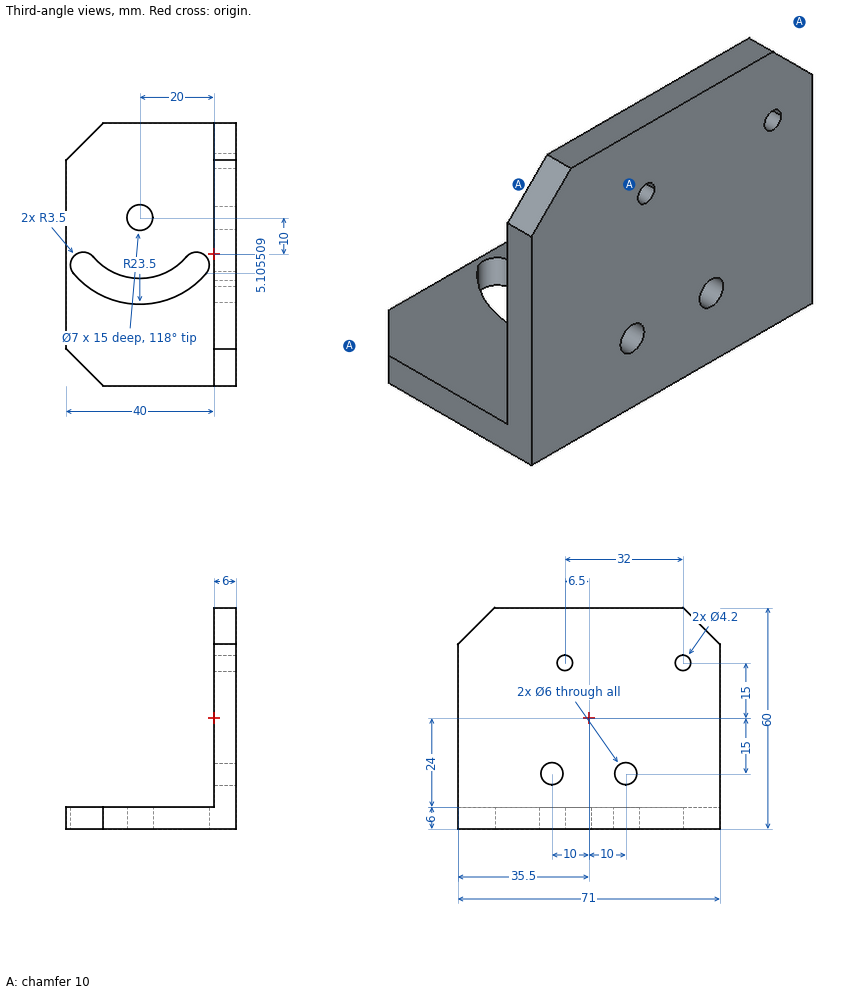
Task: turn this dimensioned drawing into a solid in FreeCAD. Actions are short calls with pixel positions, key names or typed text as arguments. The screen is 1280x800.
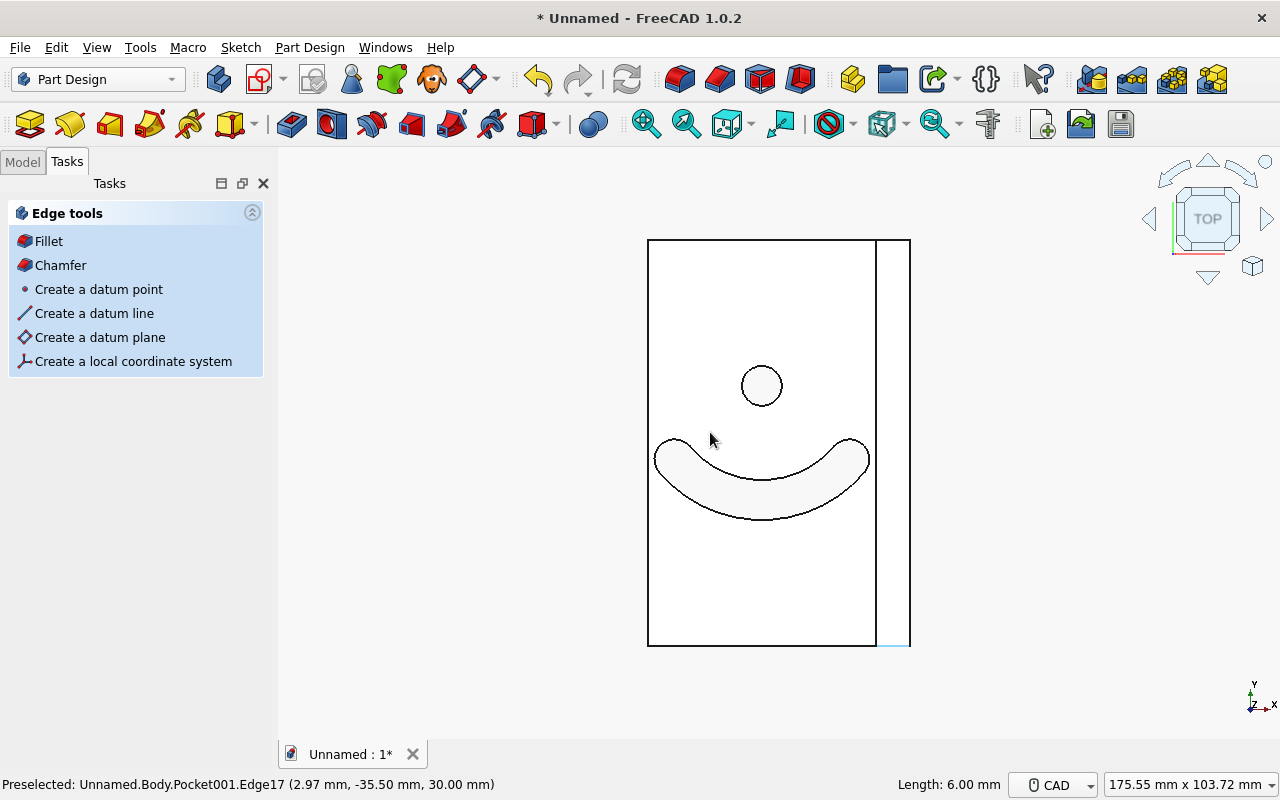
click(893, 239, ctrl)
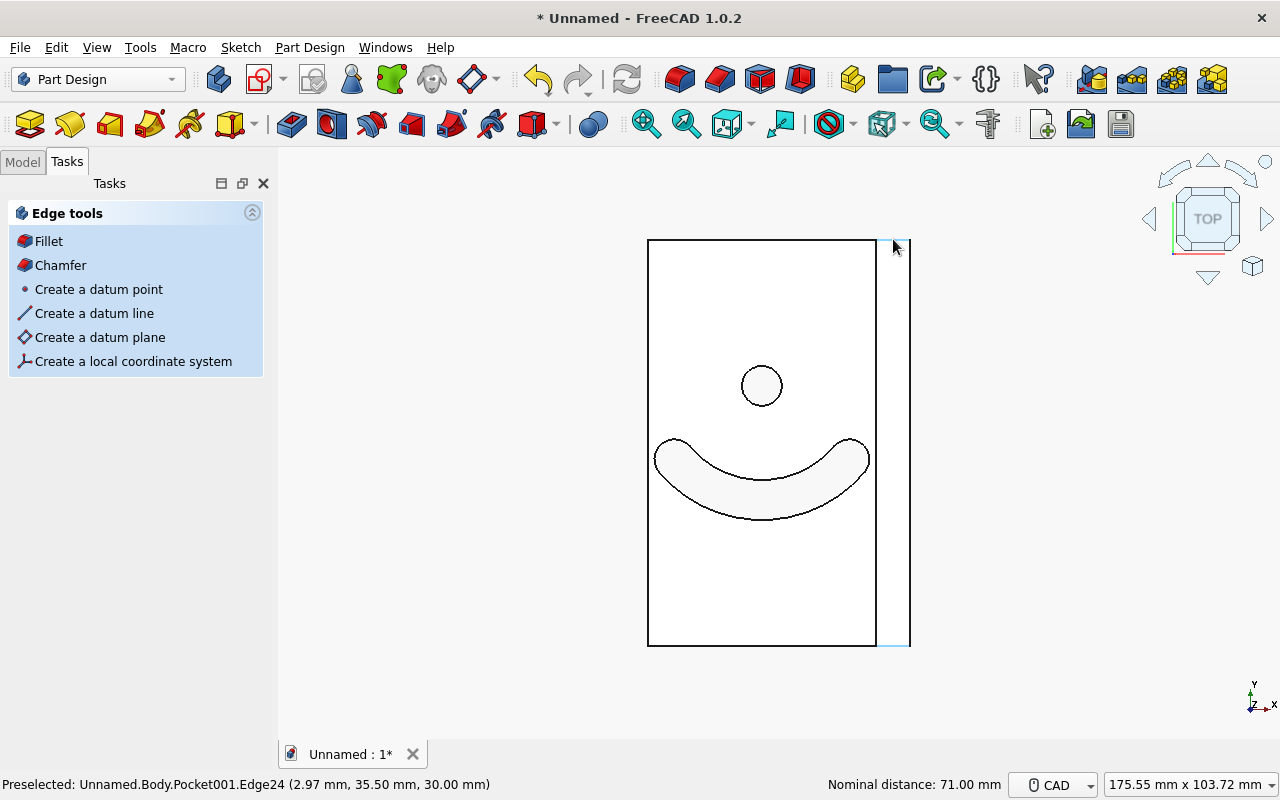
key(1)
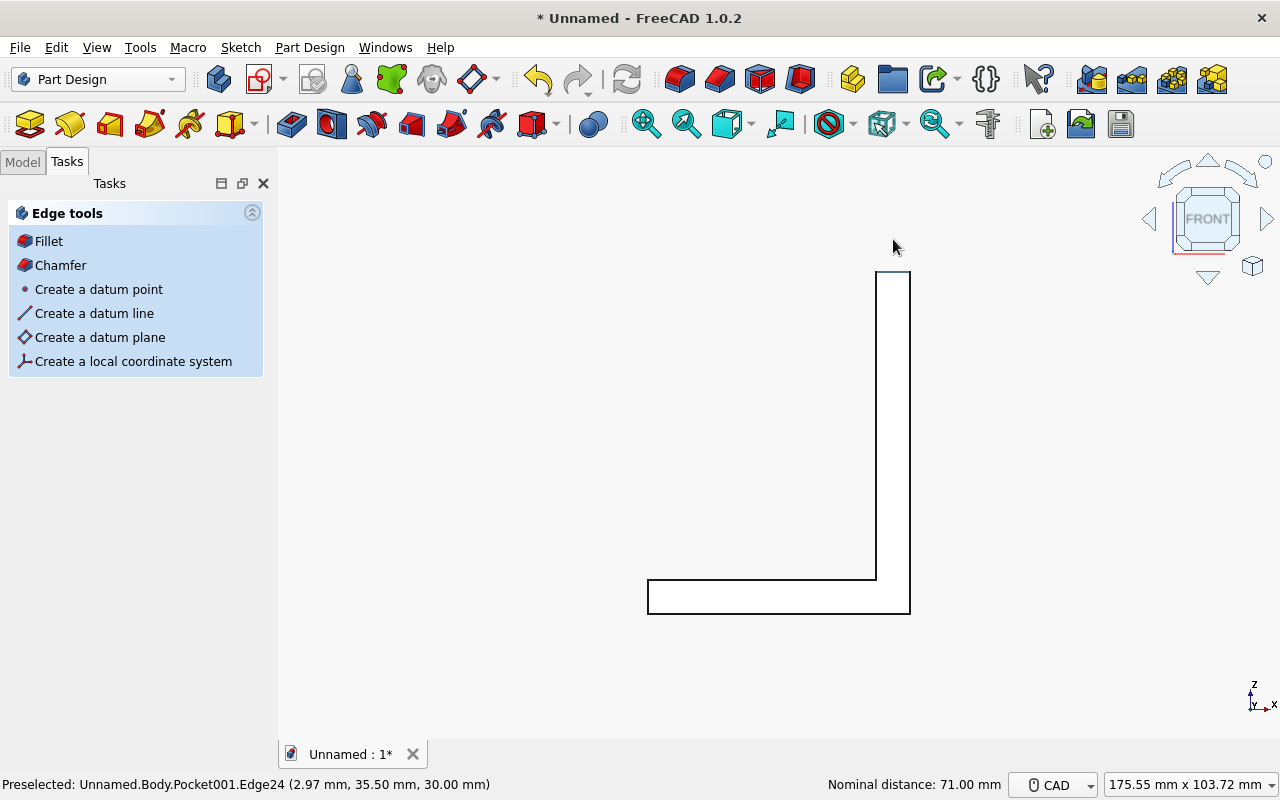
click(648, 596, ctrl)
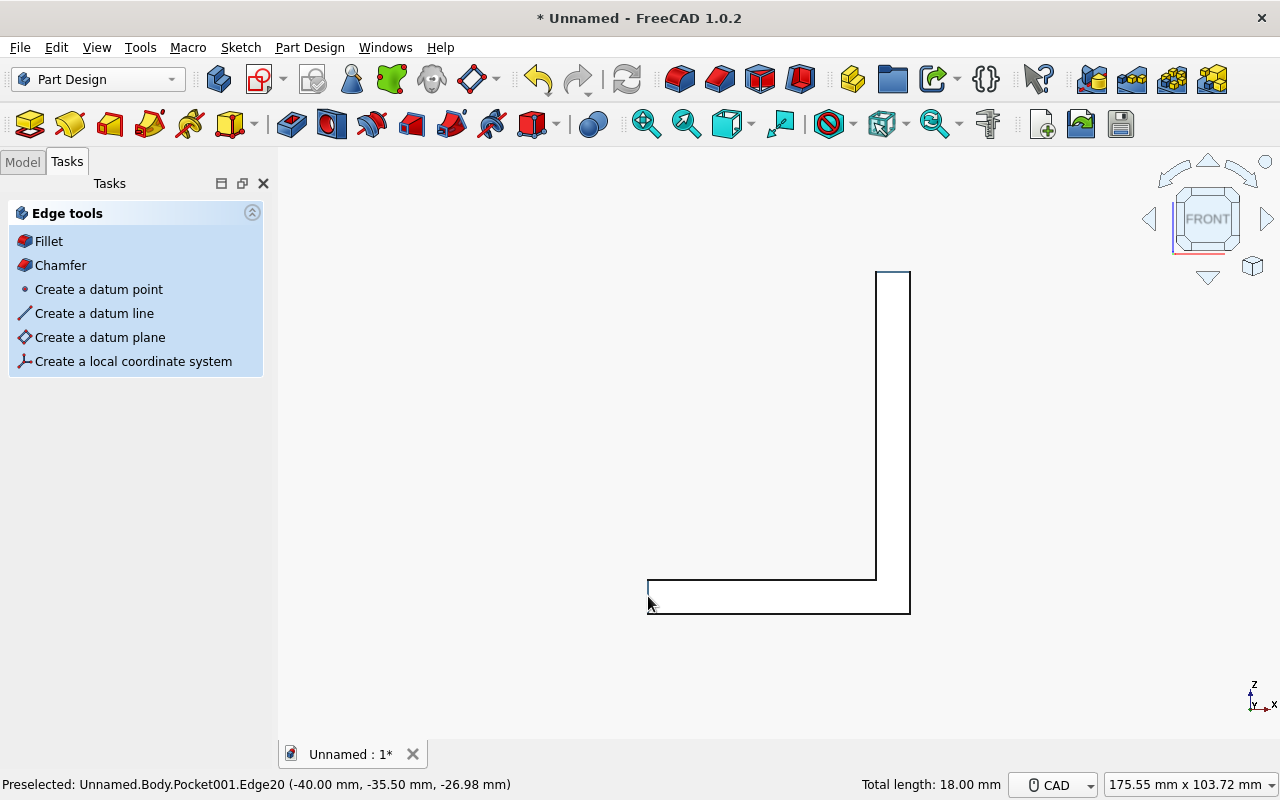
key(3)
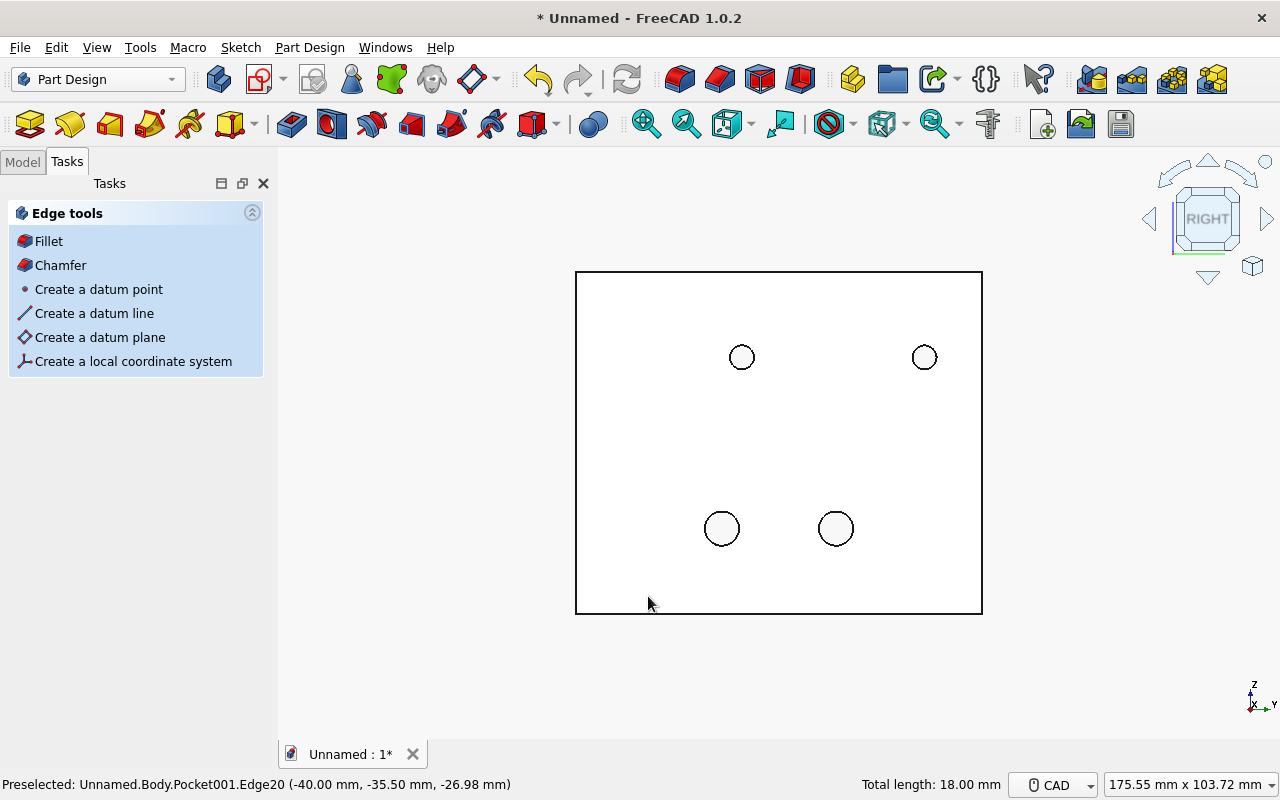
key(5)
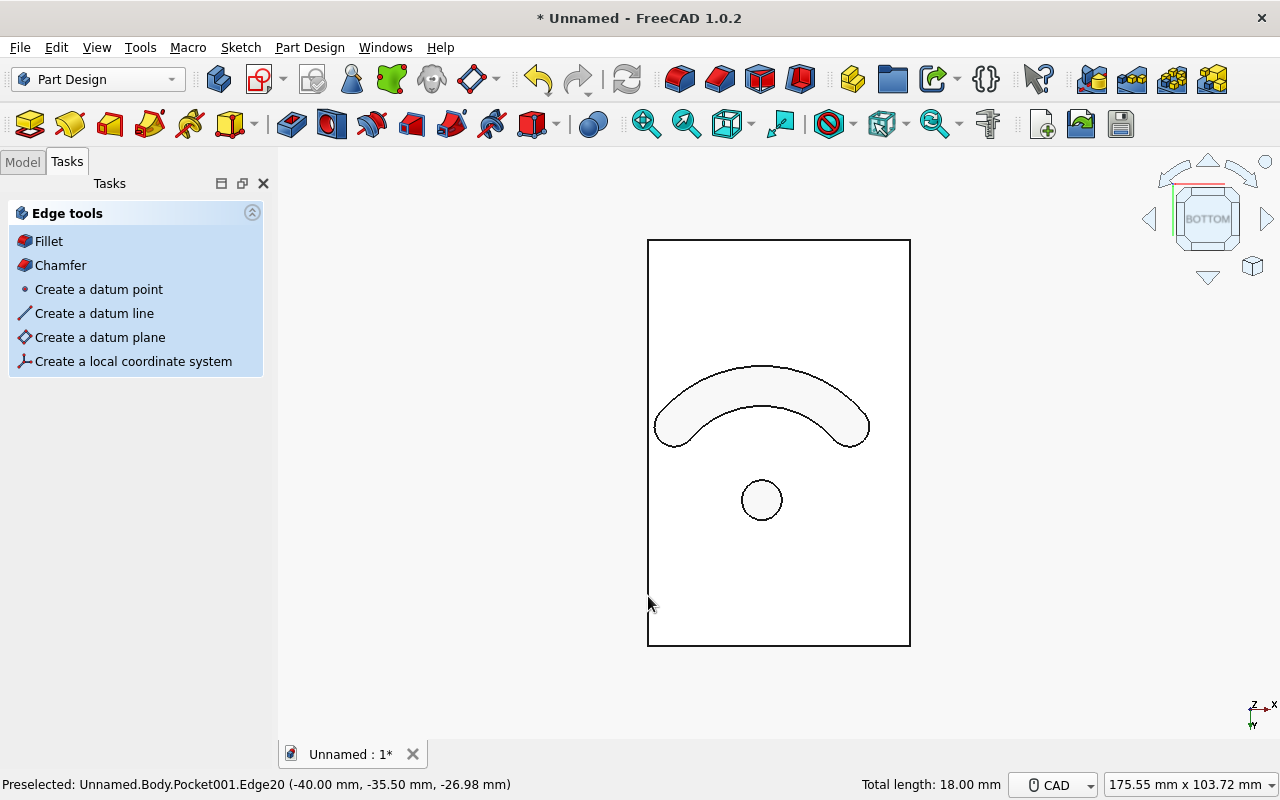
key(4)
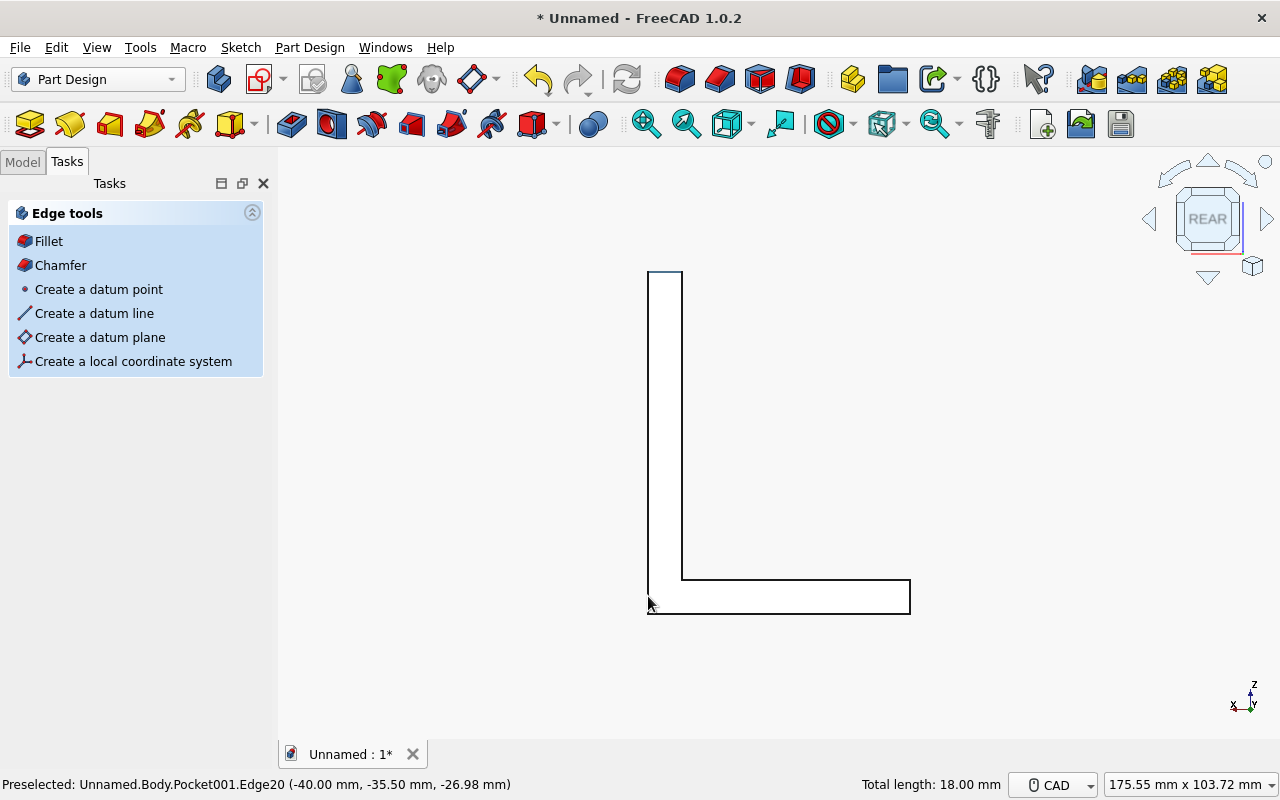
click(910, 596, ctrl)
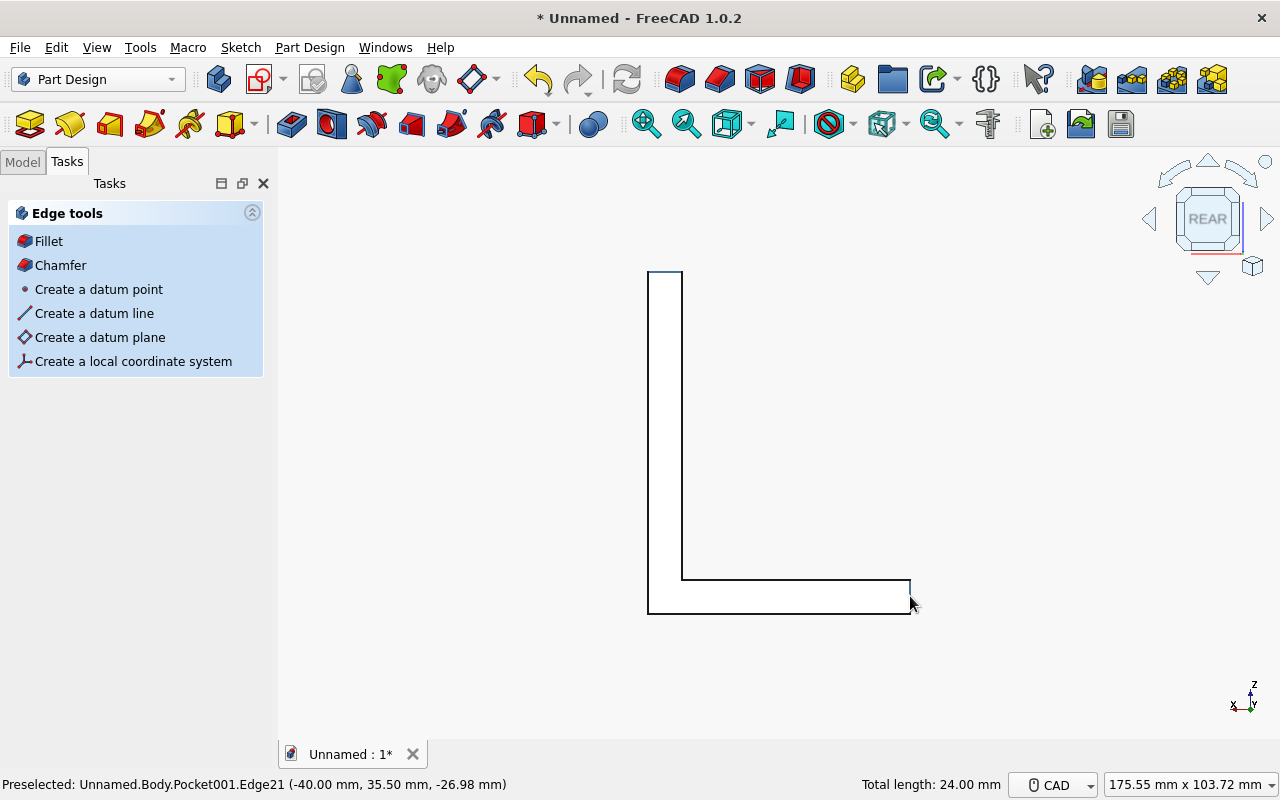
click(720, 80)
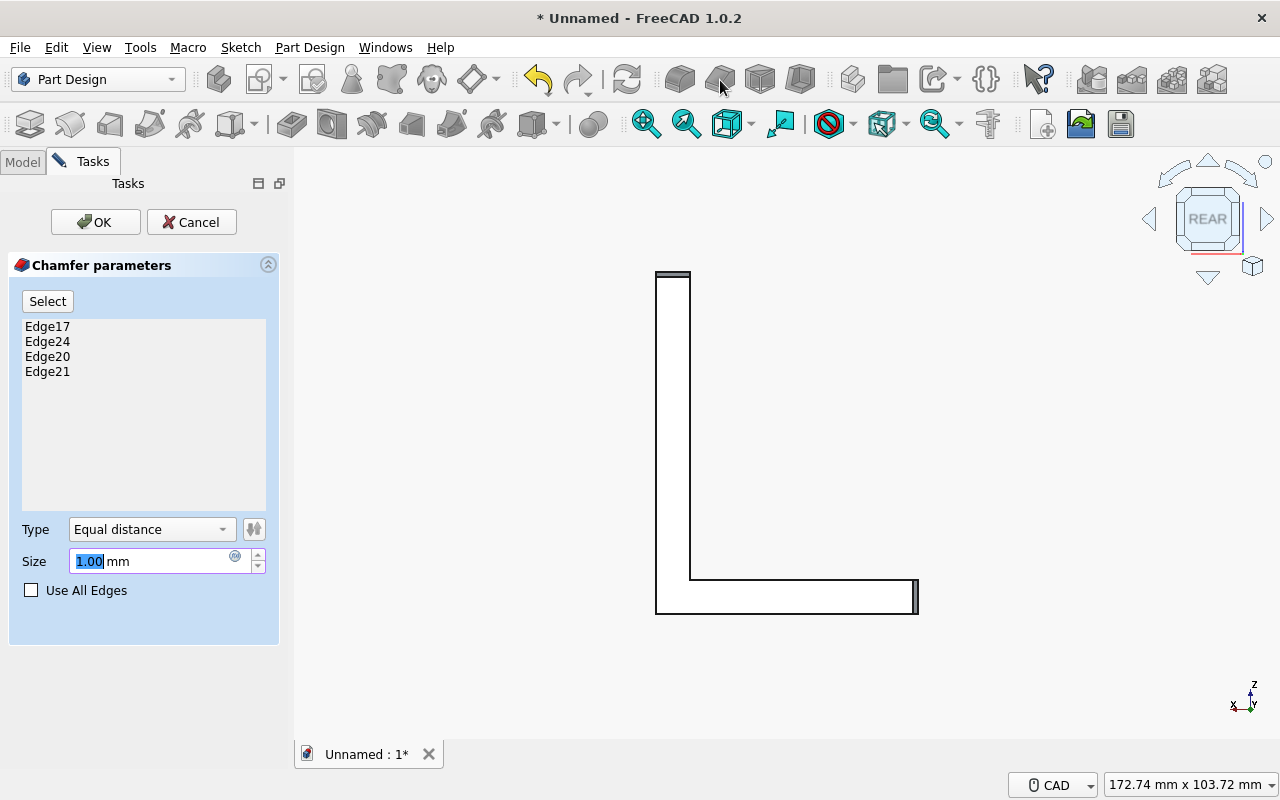
text(10)
key(Tab)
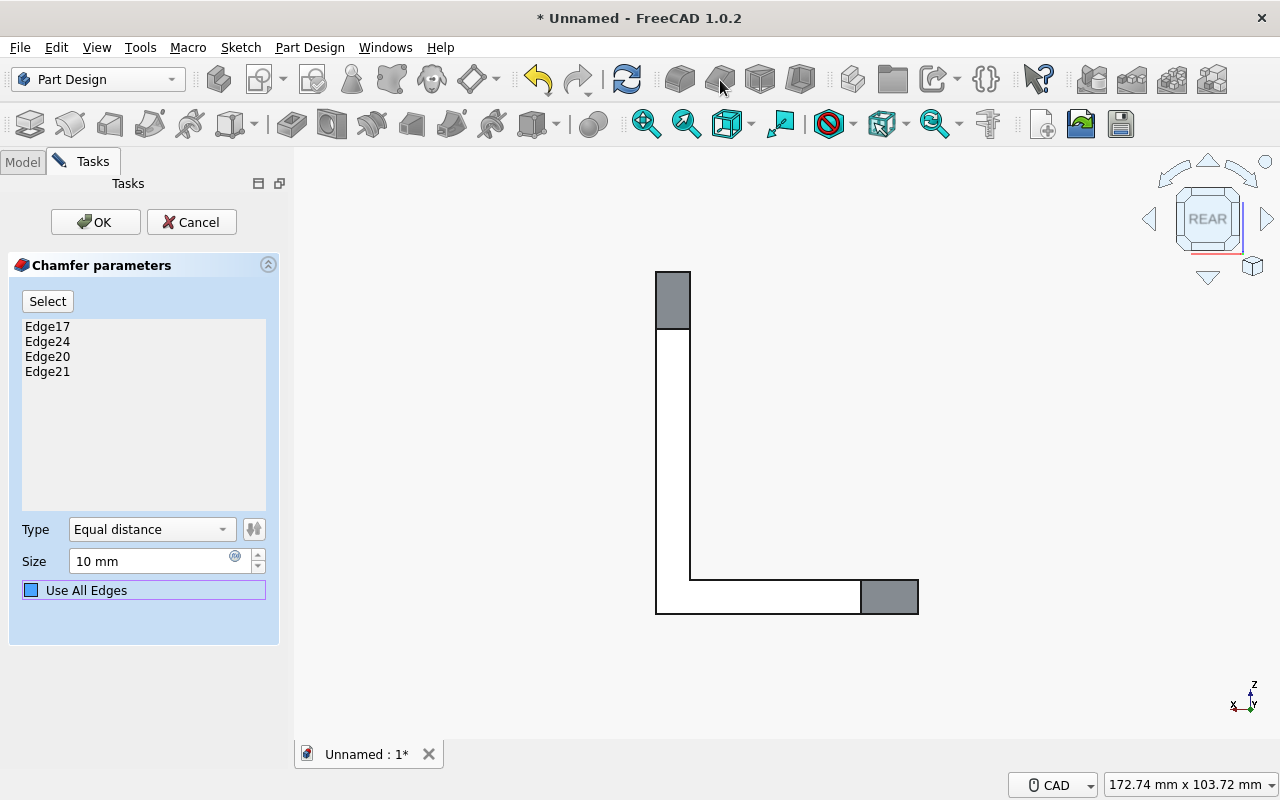
click(96, 222)